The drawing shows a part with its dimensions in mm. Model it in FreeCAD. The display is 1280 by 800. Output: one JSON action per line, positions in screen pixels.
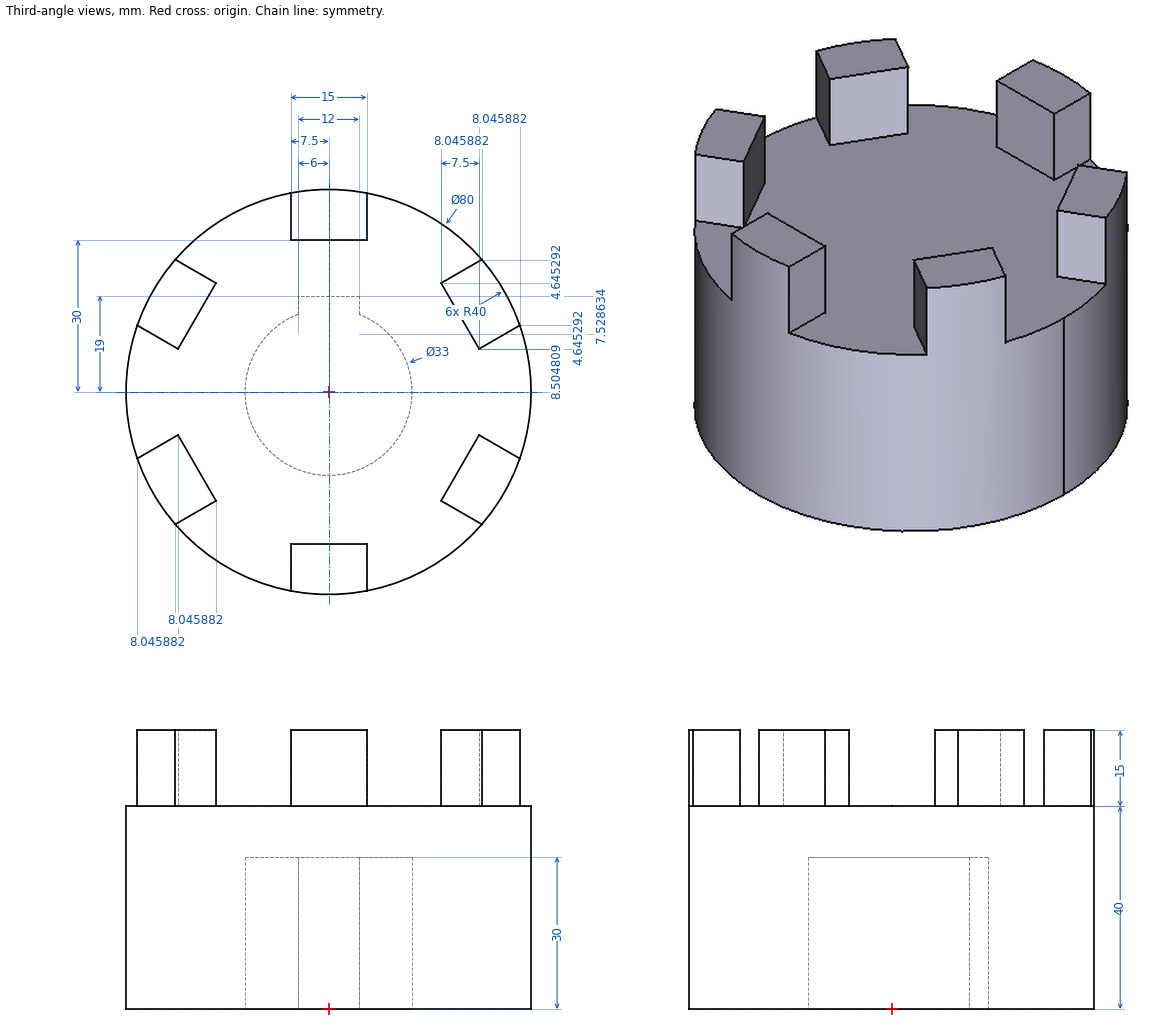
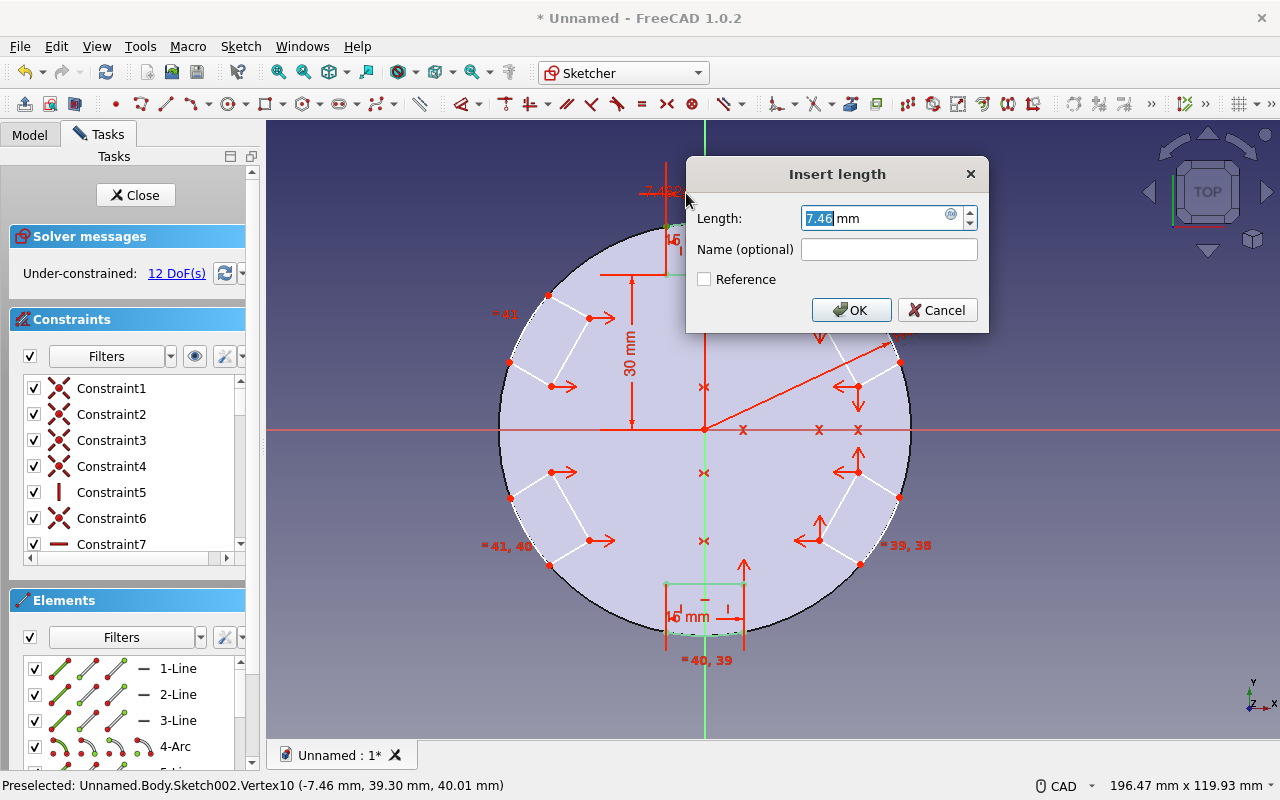
{"action": "type", "text": "7.5"}
{"action": "key", "text": "Return"}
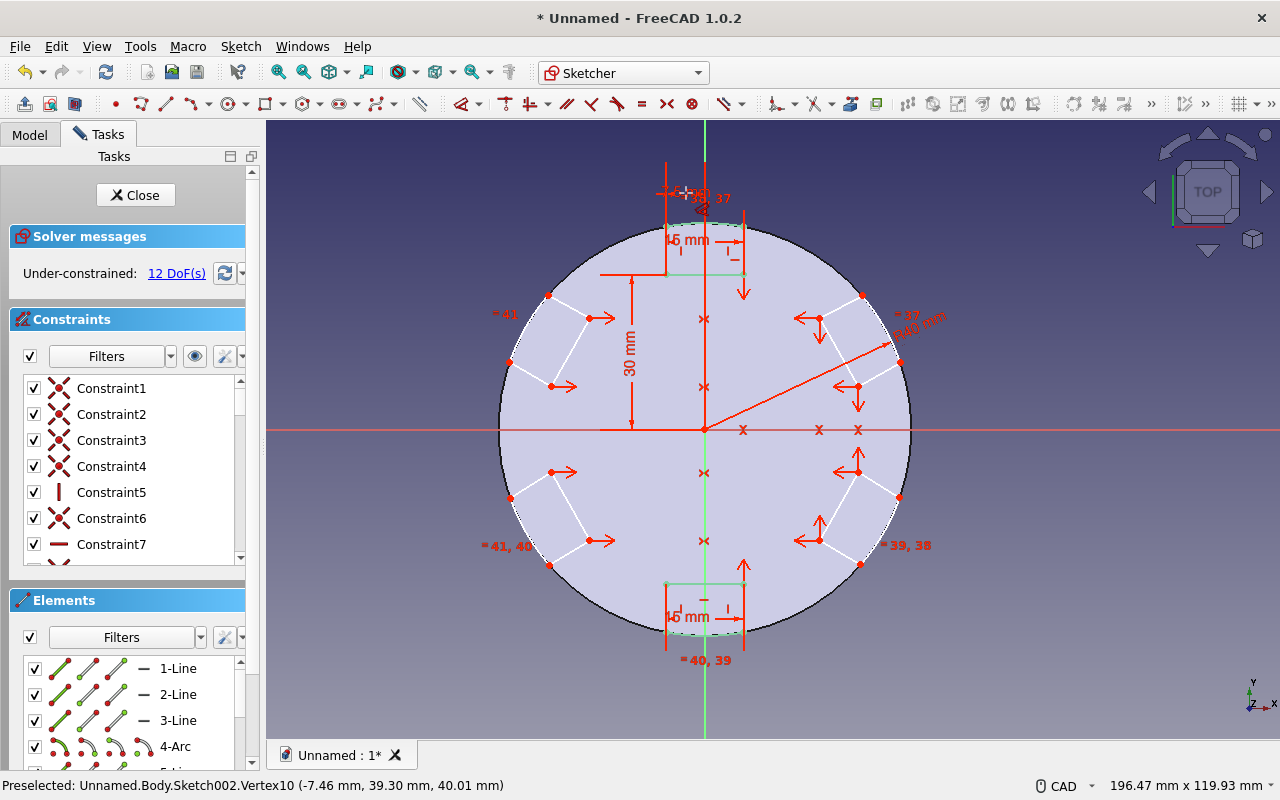
{"action": "left_click", "coordinate": [831, 339]}
{"action": "left_click", "coordinate": [839, 284]}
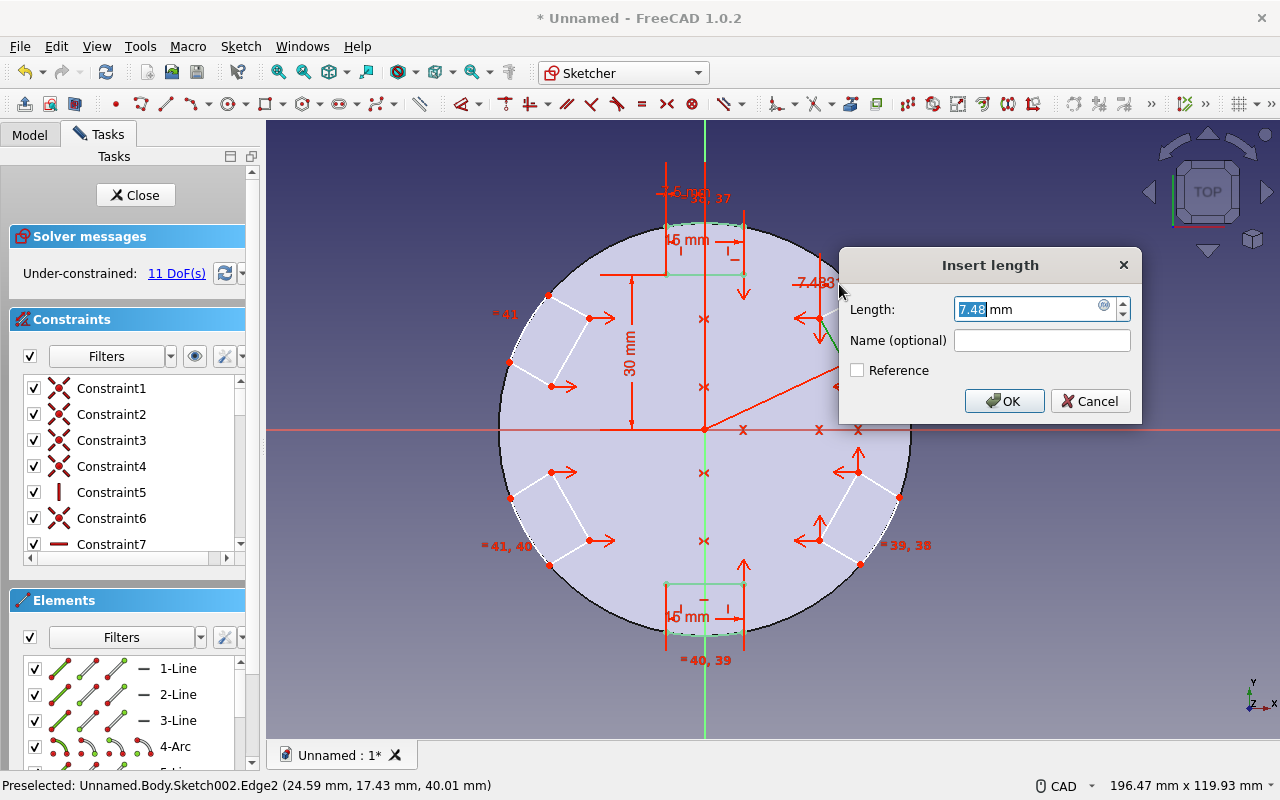
{"action": "type", "text": "7.5"}
{"action": "key", "text": "Return"}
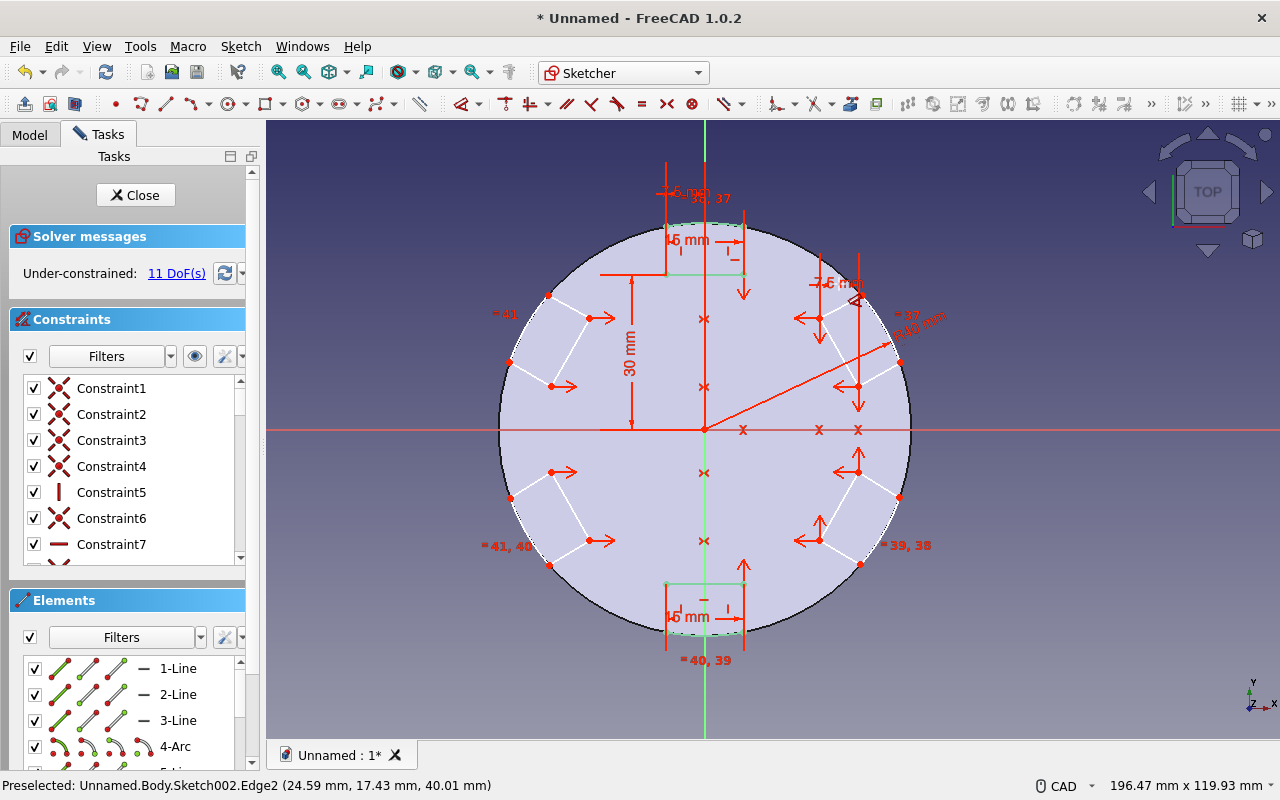
{"action": "left_click", "coordinate": [859, 387]}
{"action": "left_click", "coordinate": [893, 408]}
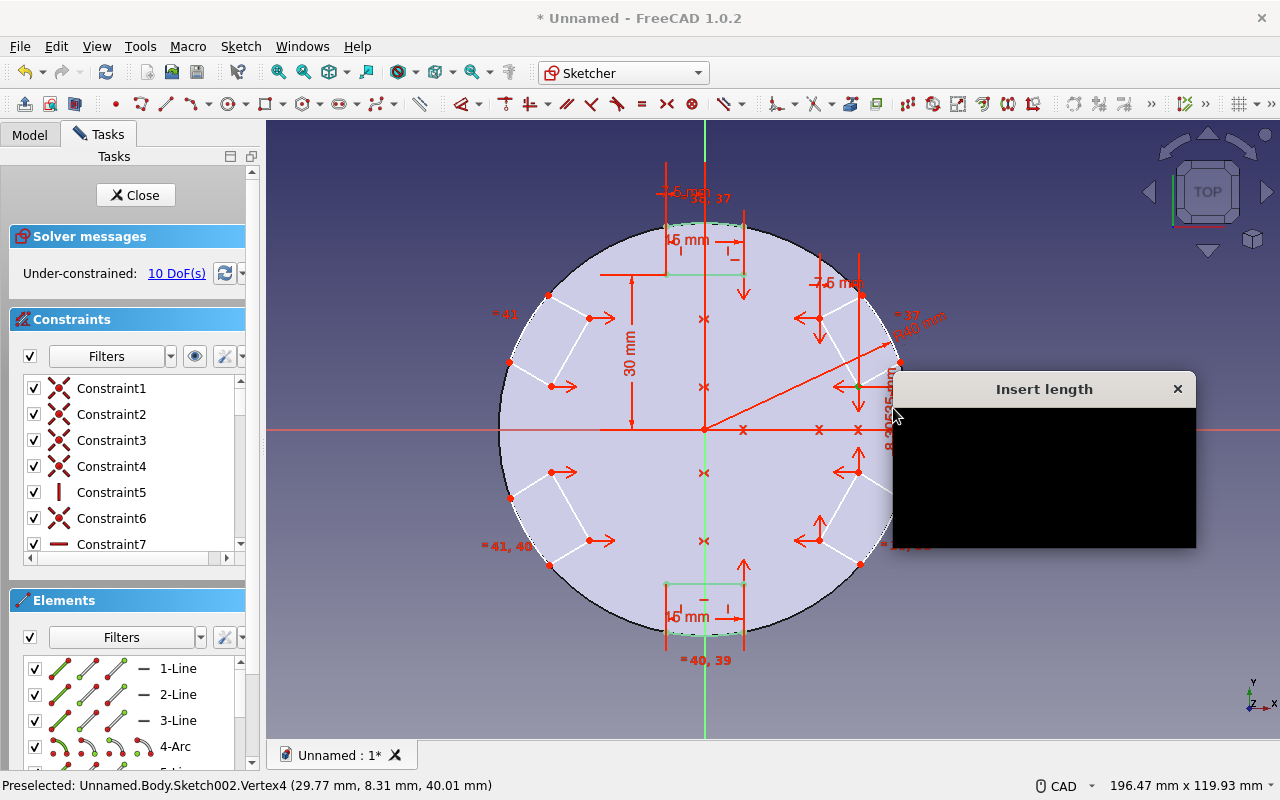
{"action": "type", "text": "8.504809"}
{"action": "key", "text": "Return"}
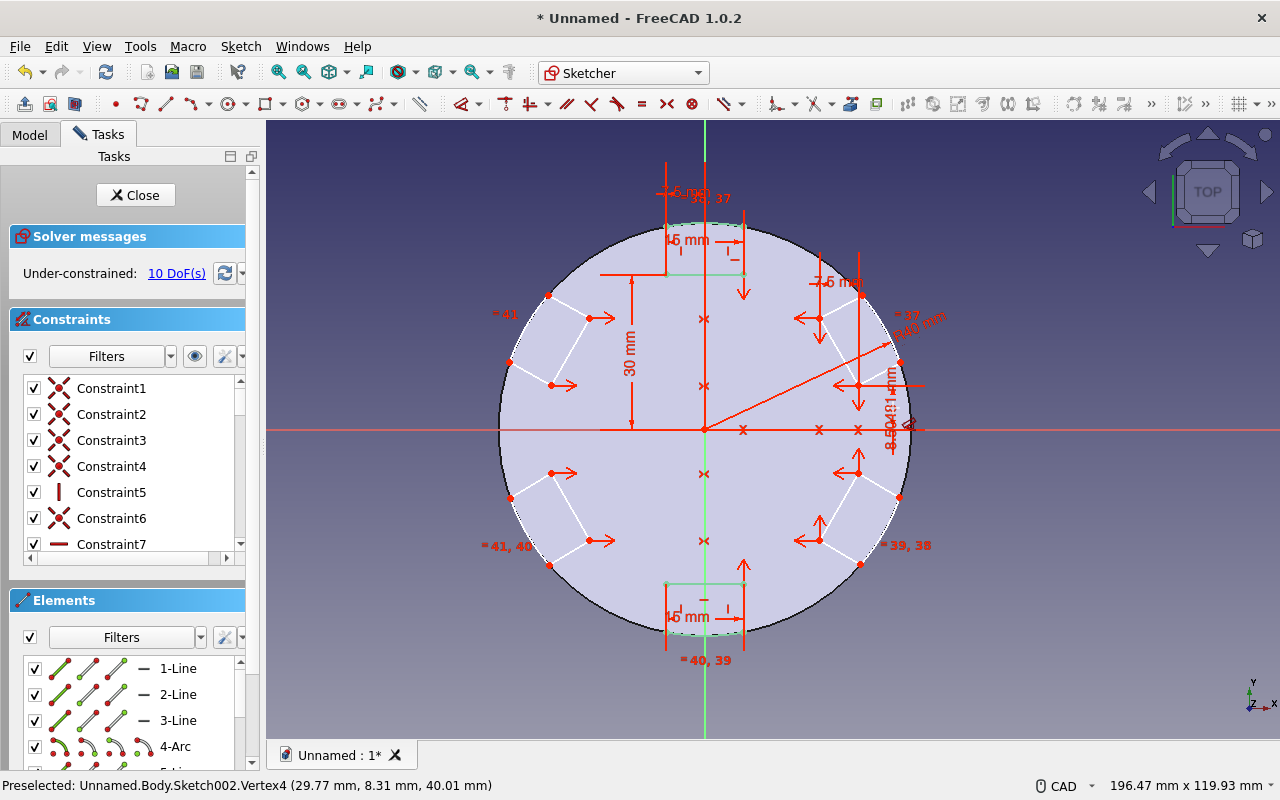
{"action": "left_click", "coordinate": [850, 303]}
{"action": "left_click", "coordinate": [841, 262]}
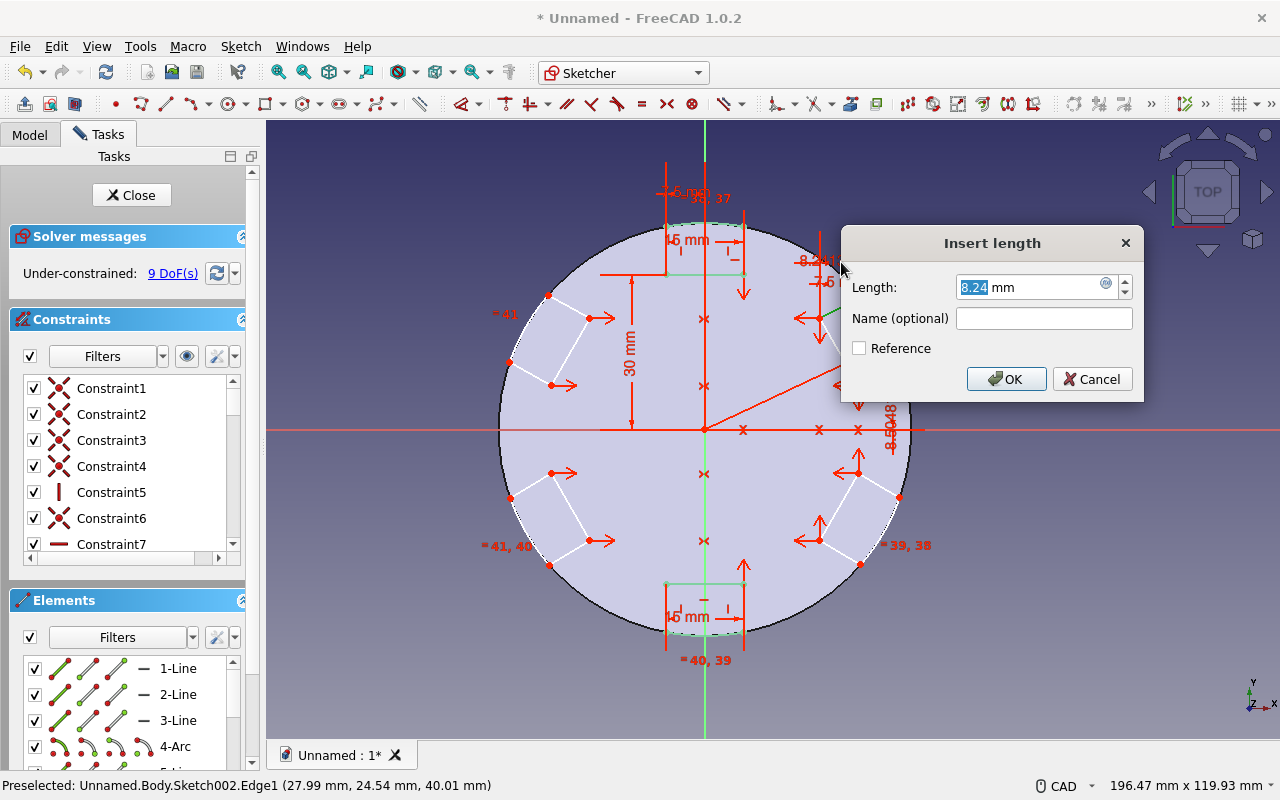
{"action": "type", "text": "8.045882"}
{"action": "key", "text": "Return"}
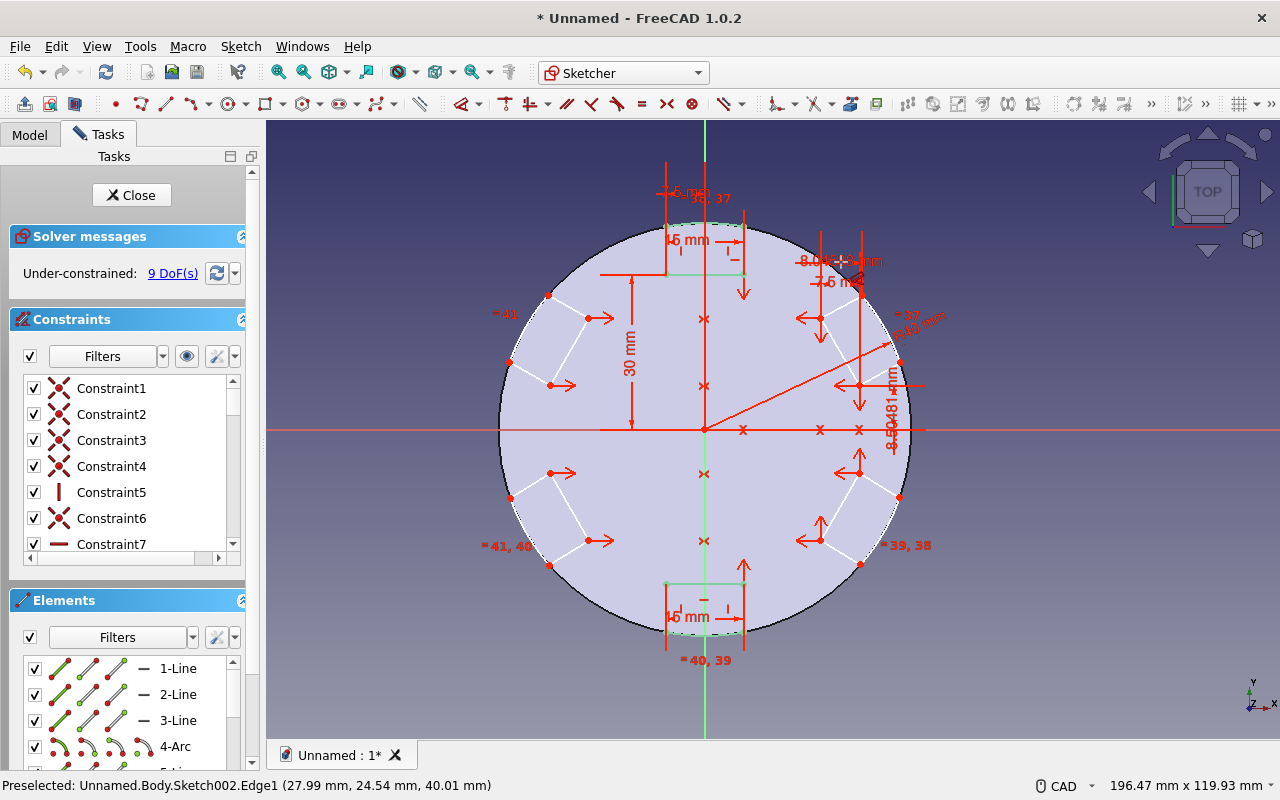
{"action": "scroll", "coordinate": [850, 303], "scroll_direction": "up", "scroll_amount": 3}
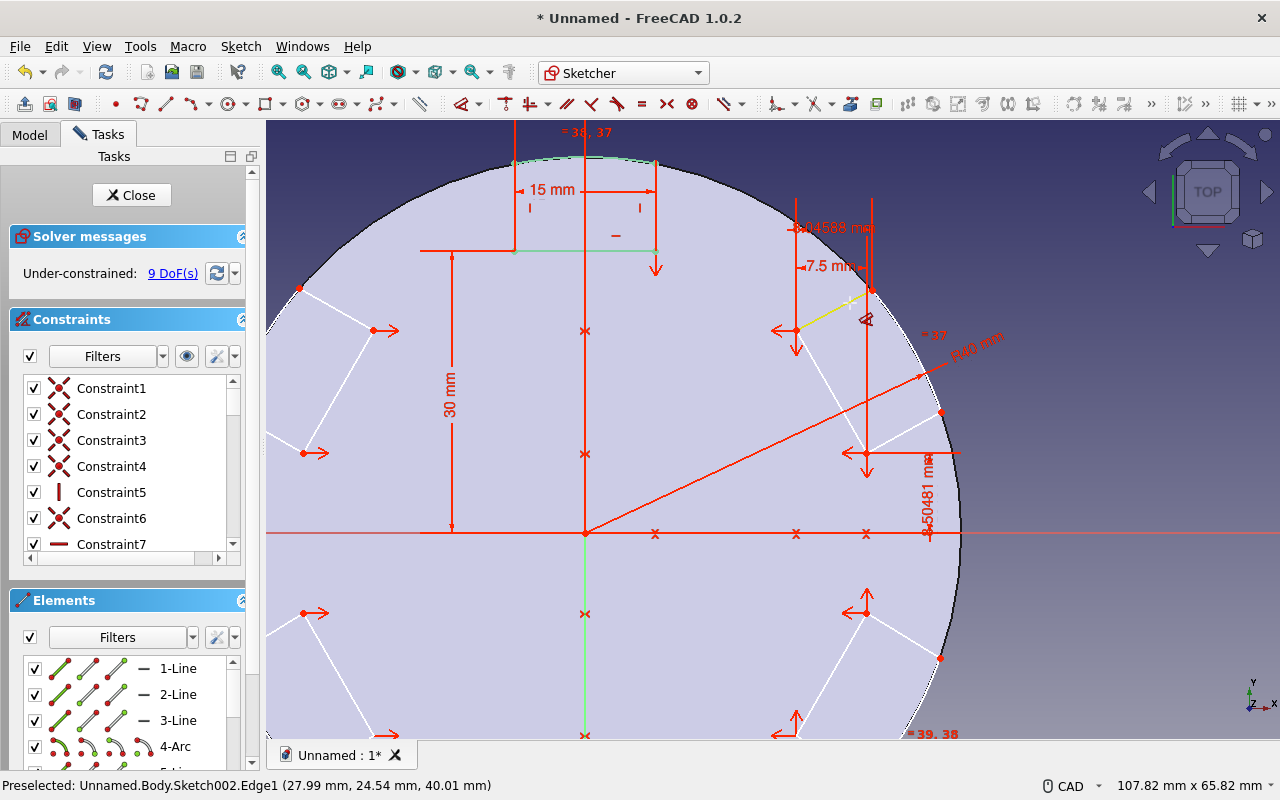
{"action": "left_click", "coordinate": [849, 302]}
{"action": "left_click", "coordinate": [906, 310]}